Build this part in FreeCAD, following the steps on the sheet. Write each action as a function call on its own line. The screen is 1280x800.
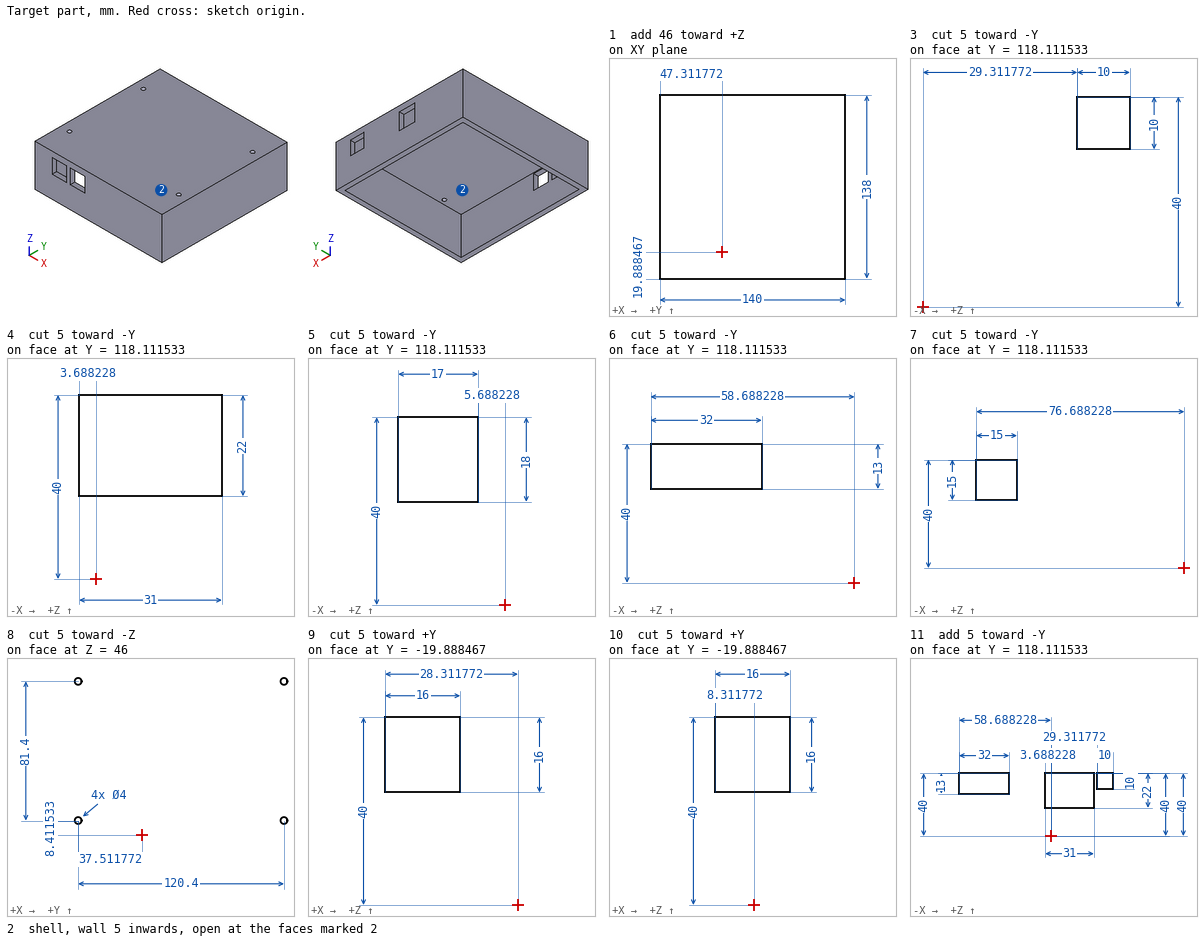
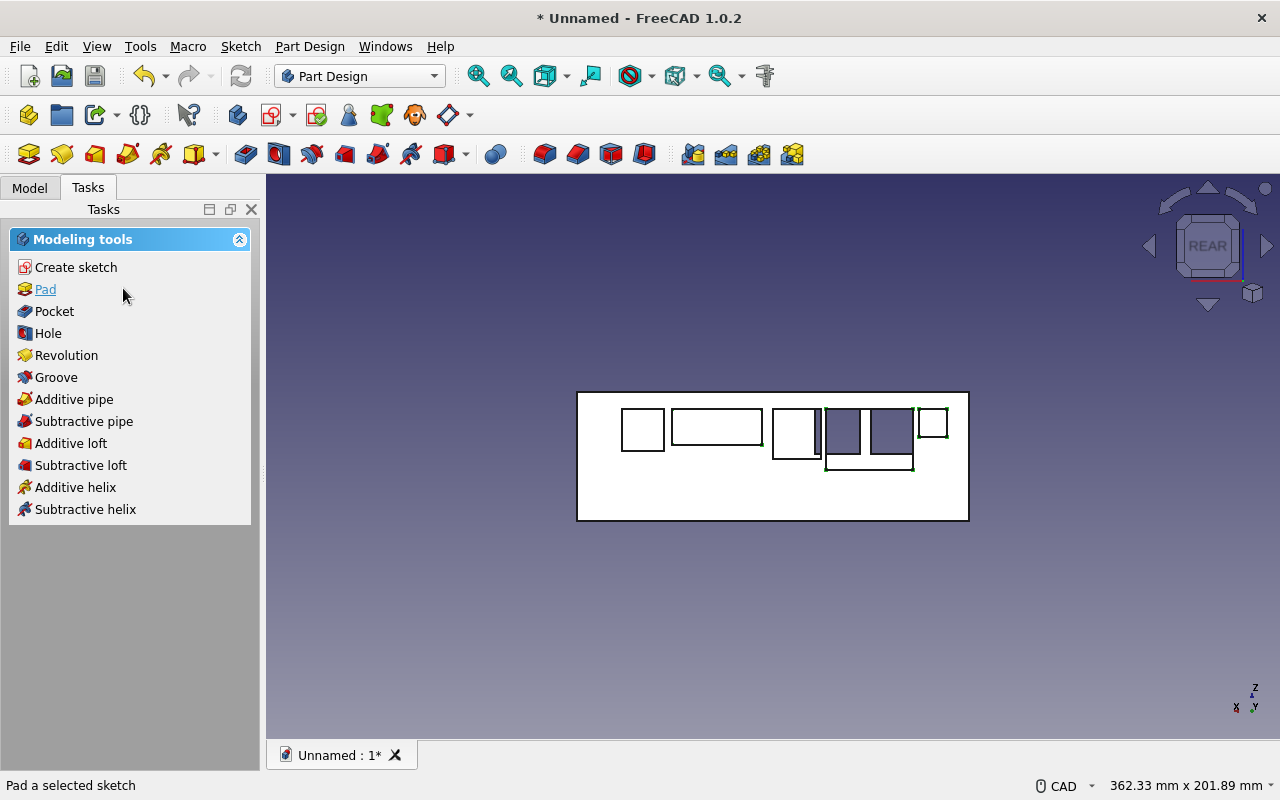
click(29, 154)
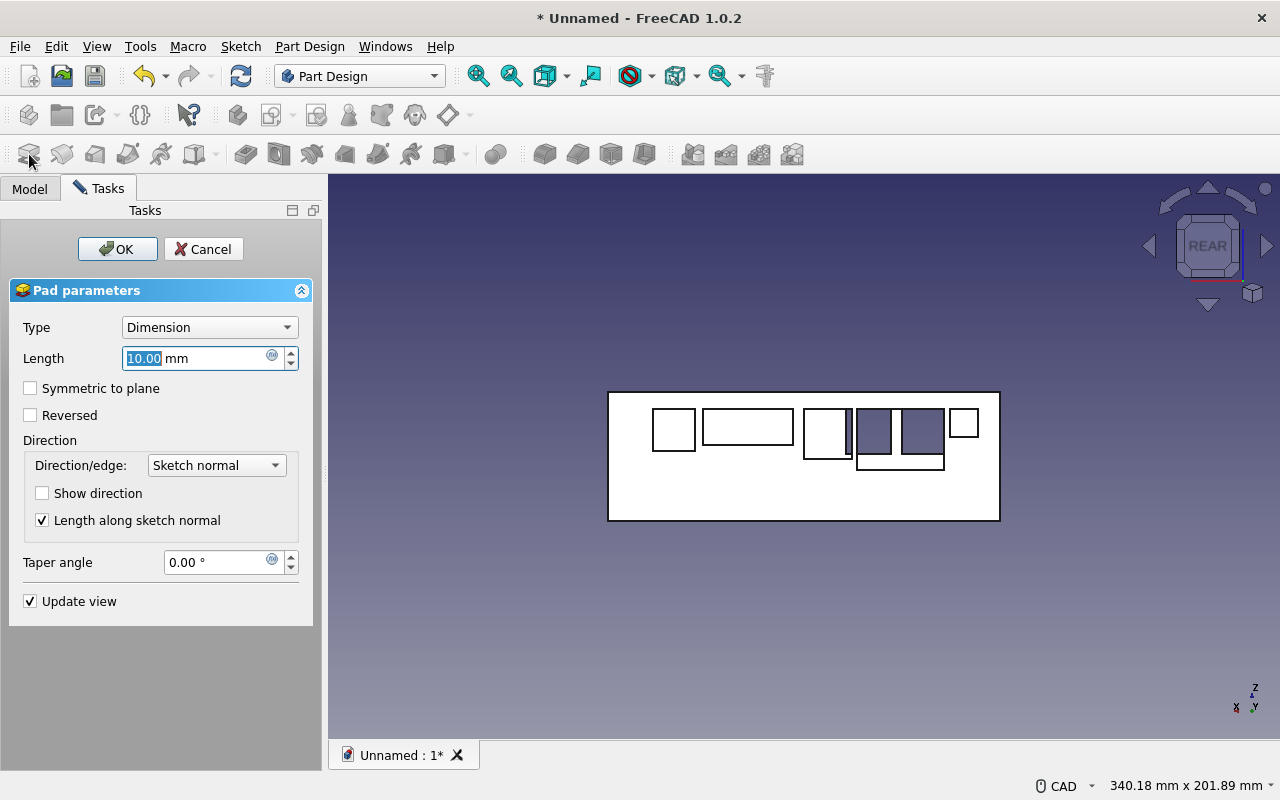
text(5)
key(Tab)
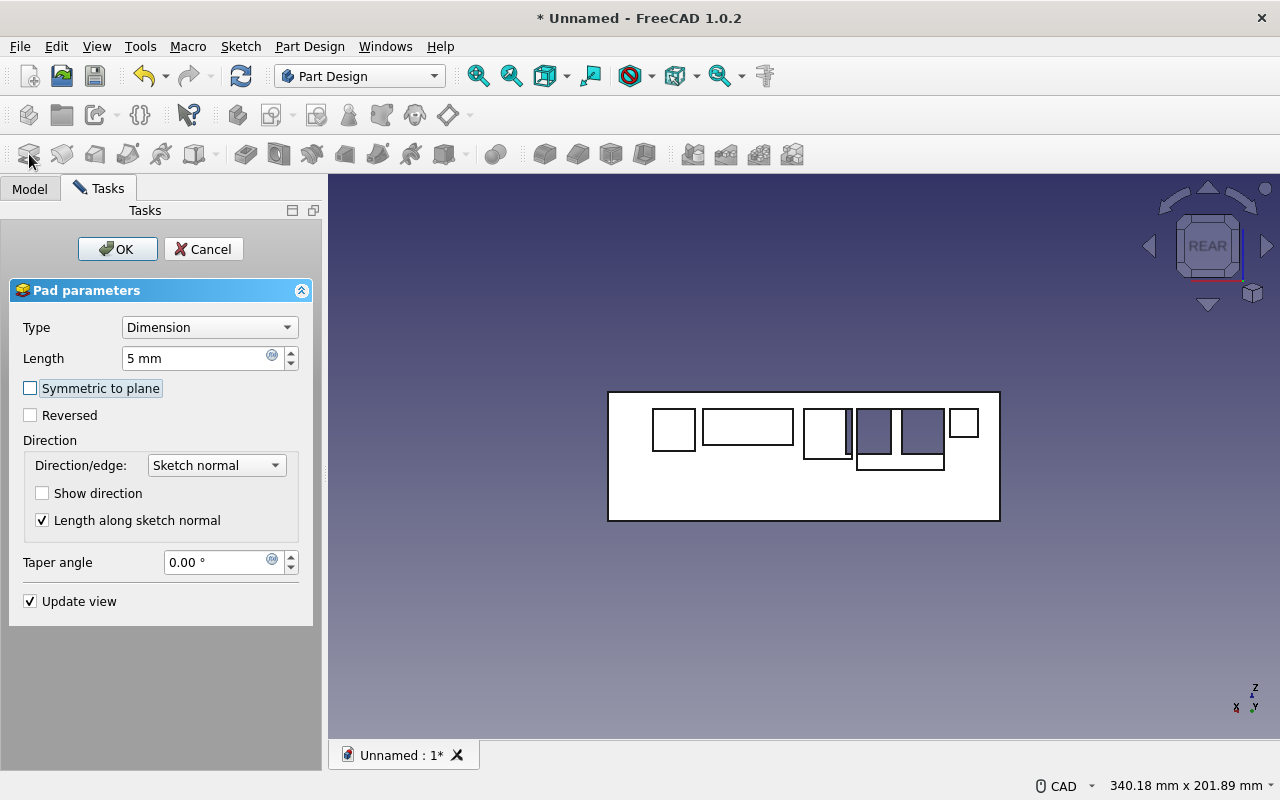
click(31, 415)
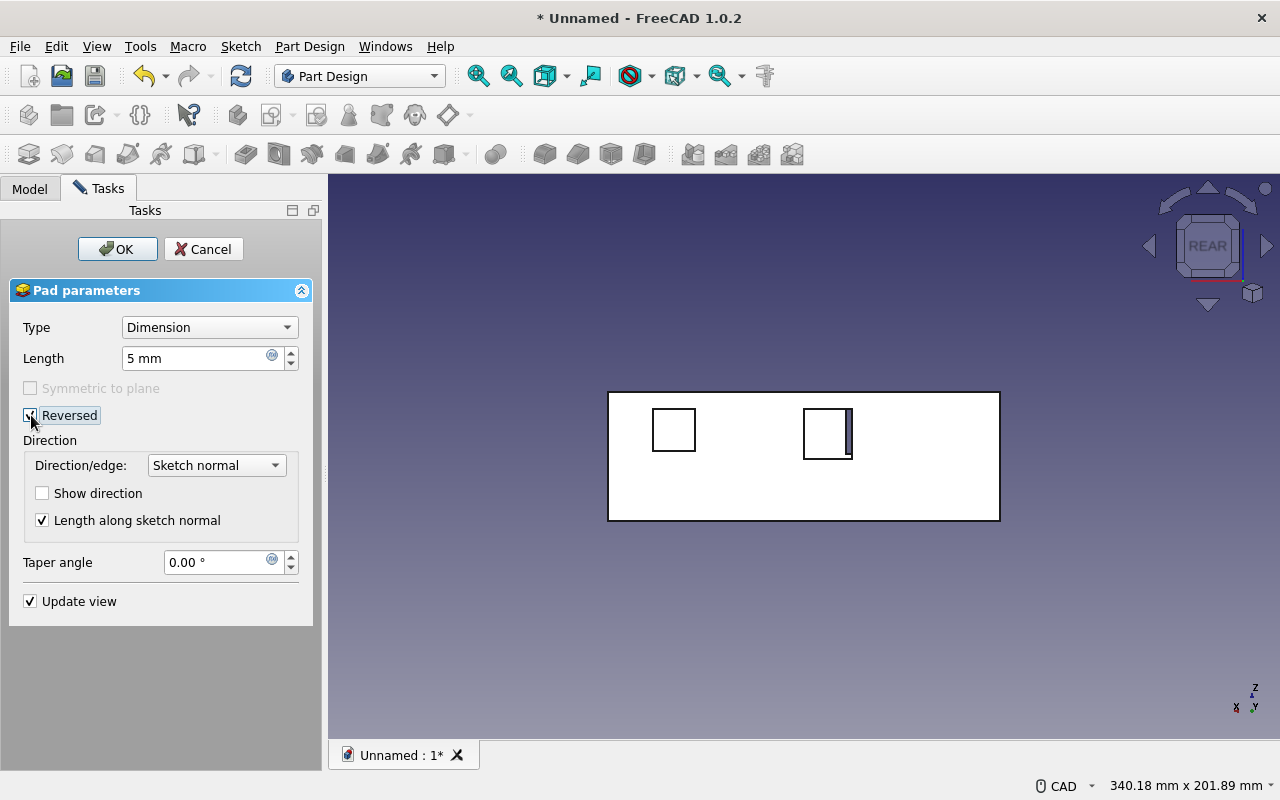
click(118, 249)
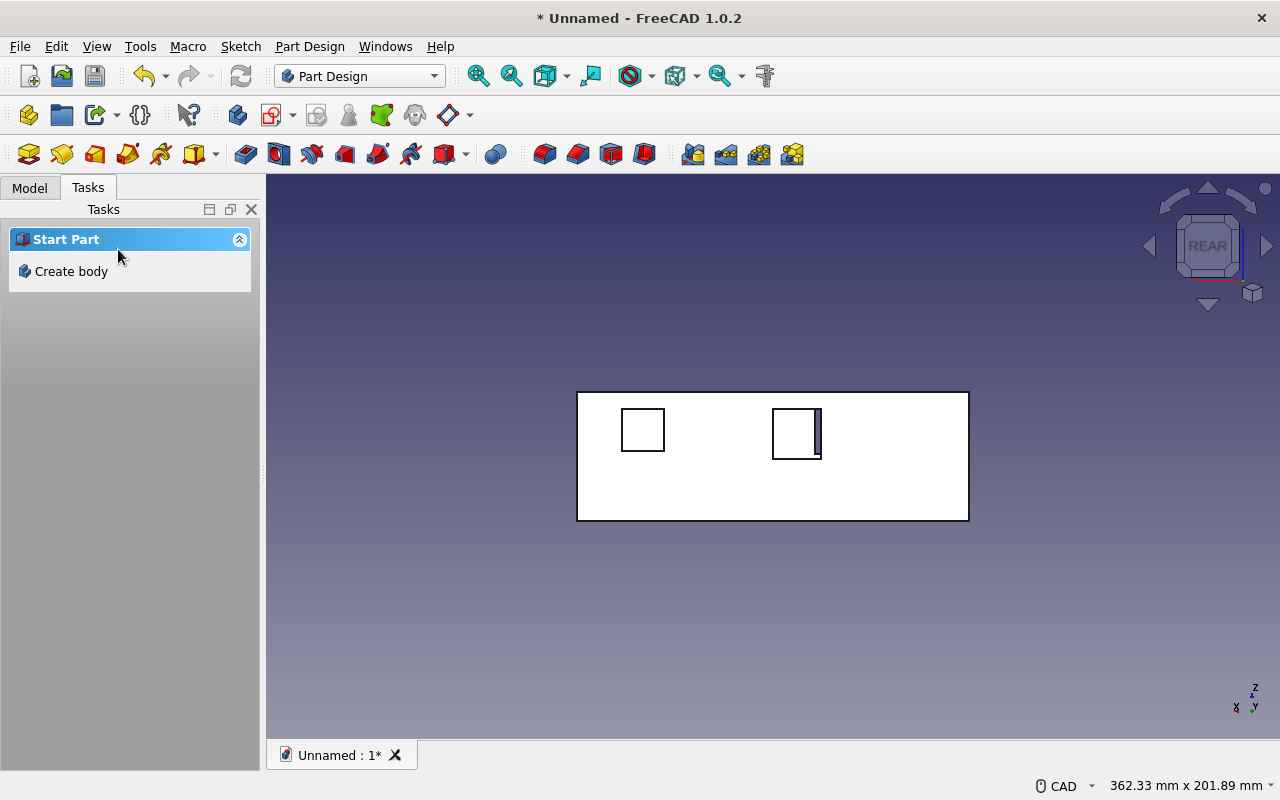
key(0)